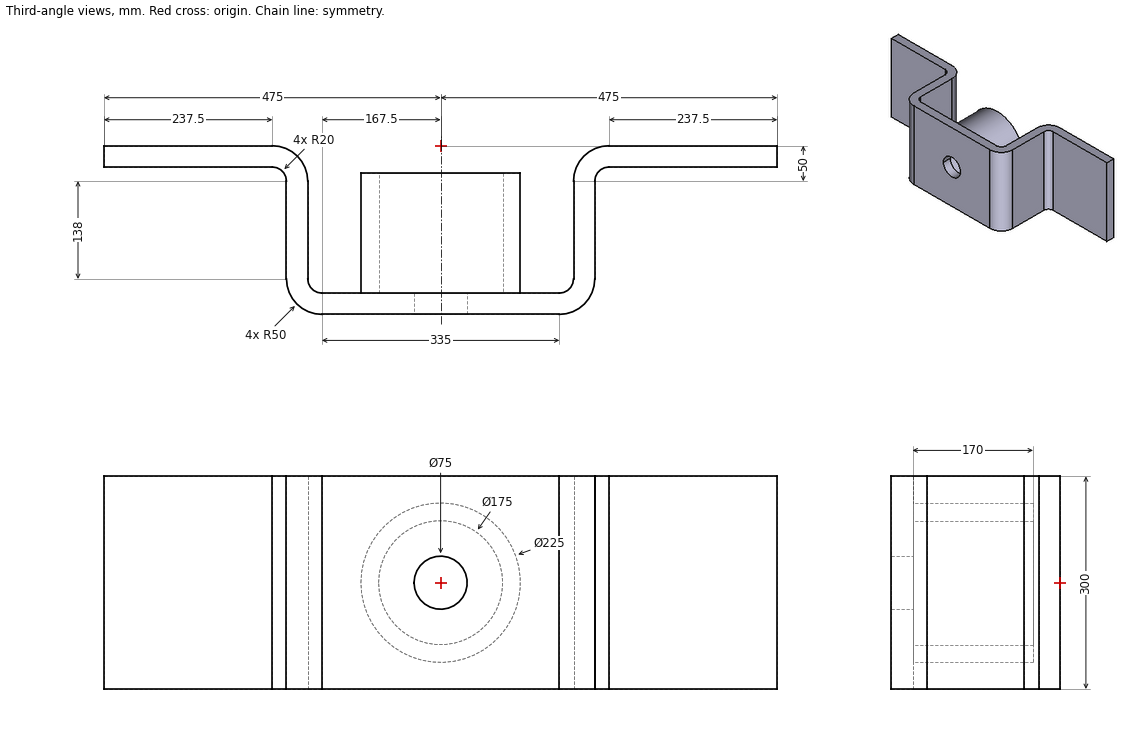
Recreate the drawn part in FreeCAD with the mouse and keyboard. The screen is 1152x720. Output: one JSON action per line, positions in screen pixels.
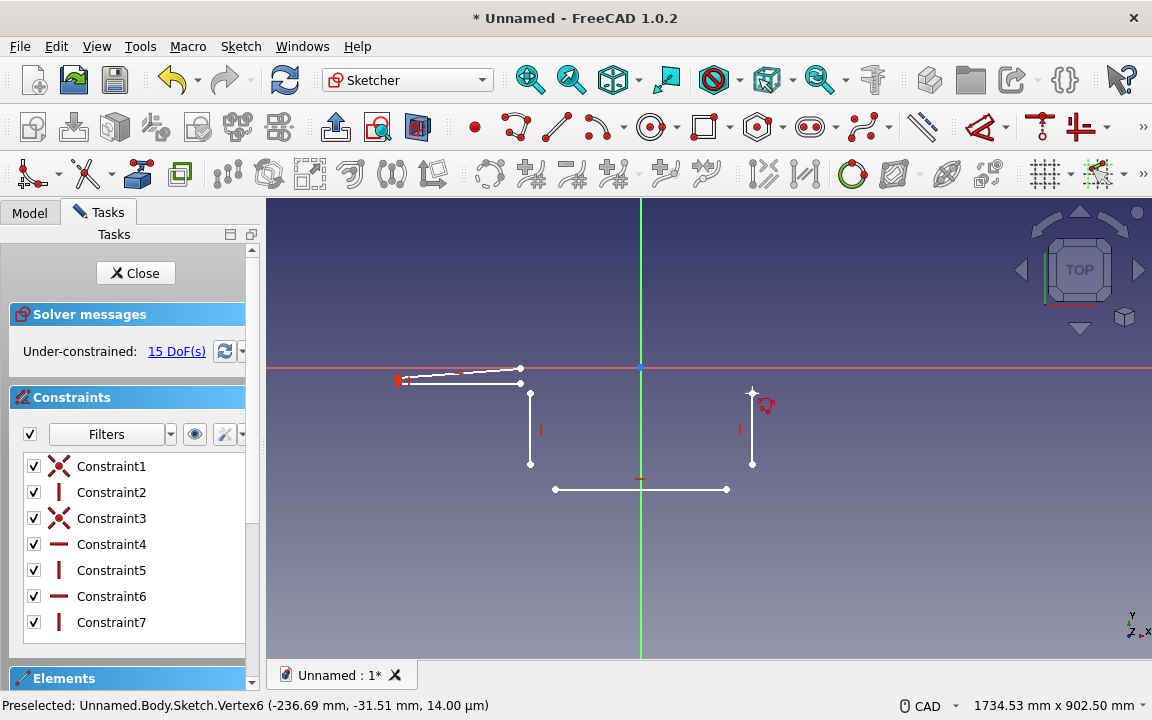
{"action": "left_click", "coordinate": [762, 383]}
{"action": "left_click", "coordinate": [884, 383]}
{"action": "left_click", "coordinate": [884, 368]}
{"action": "left_click", "coordinate": [762, 377]}
{"action": "right_click", "coordinate": [762, 377]}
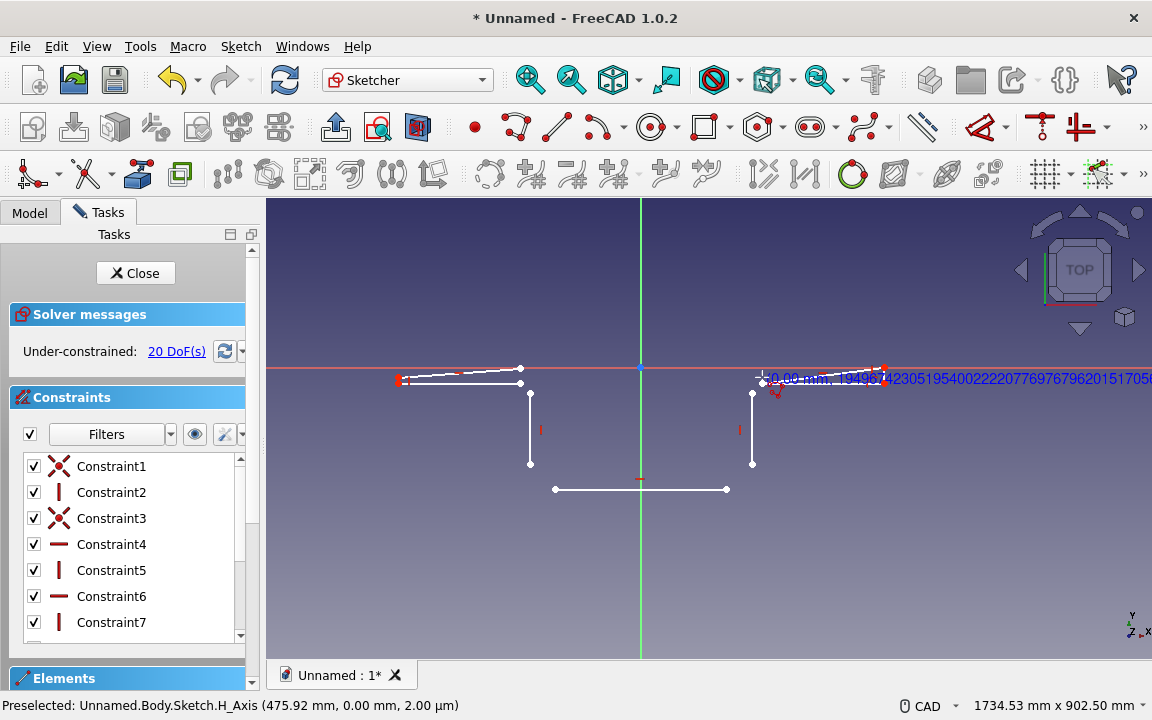
{"action": "key", "text": "g l"}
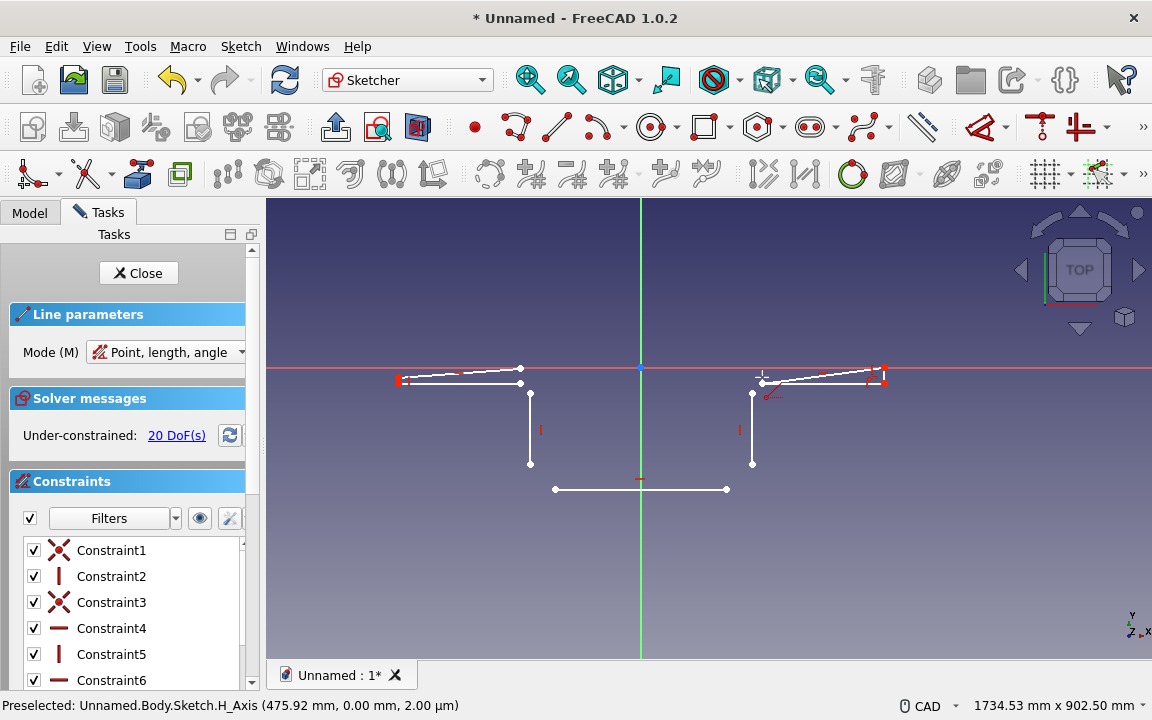
{"action": "left_click", "coordinate": [737, 393]}
{"action": "left_click", "coordinate": [737, 464]}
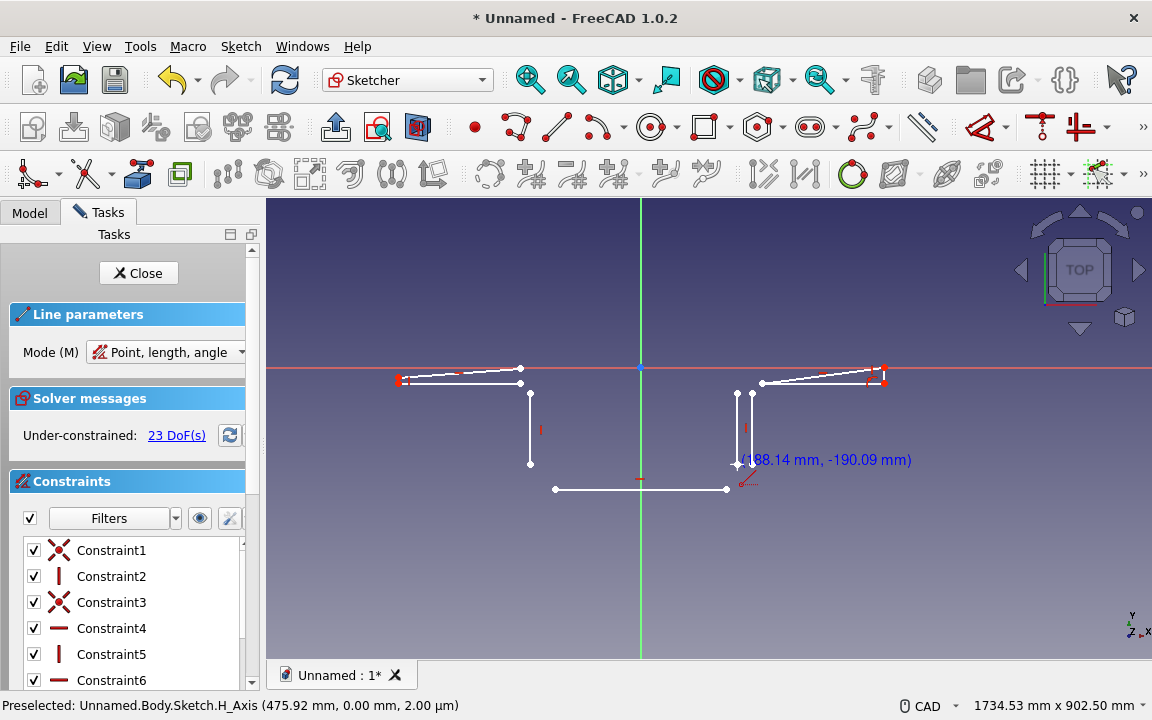
{"action": "left_click", "coordinate": [726, 474]}
{"action": "left_click", "coordinate": [555, 474]}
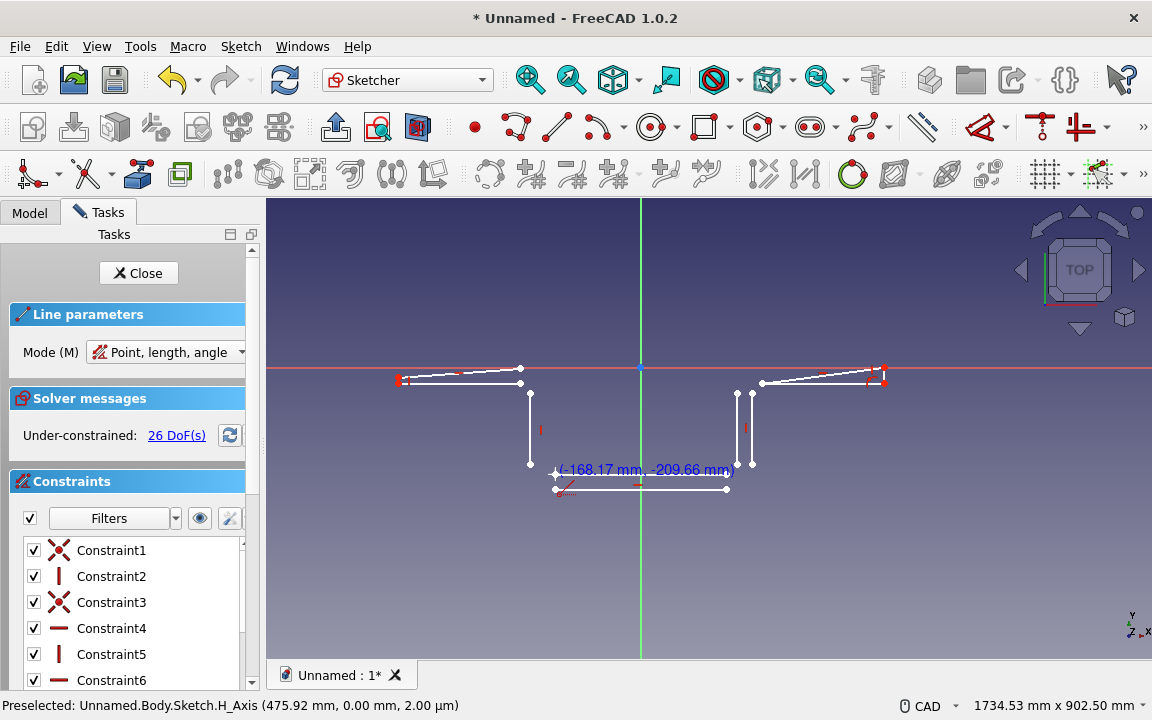
{"action": "left_click", "coordinate": [545, 464]}
{"action": "left_click", "coordinate": [545, 393]}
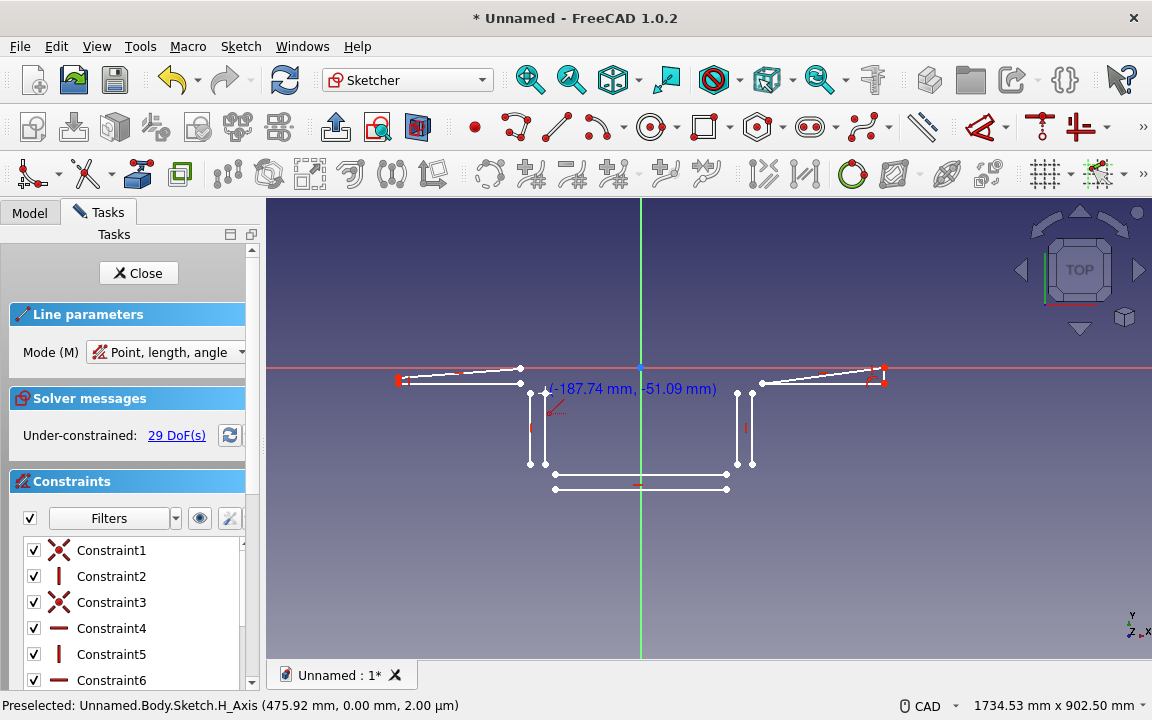
{"action": "key", "text": "g 3 a"}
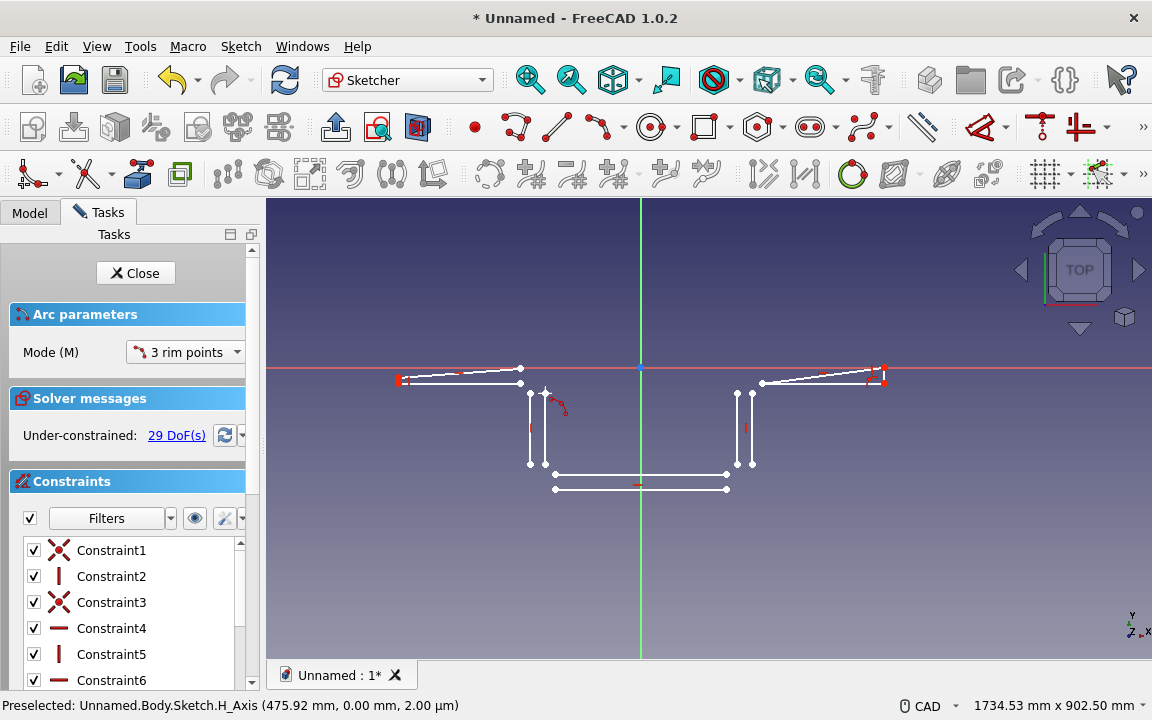
{"action": "left_click", "coordinate": [520, 384]}
{"action": "left_click", "coordinate": [530, 394]}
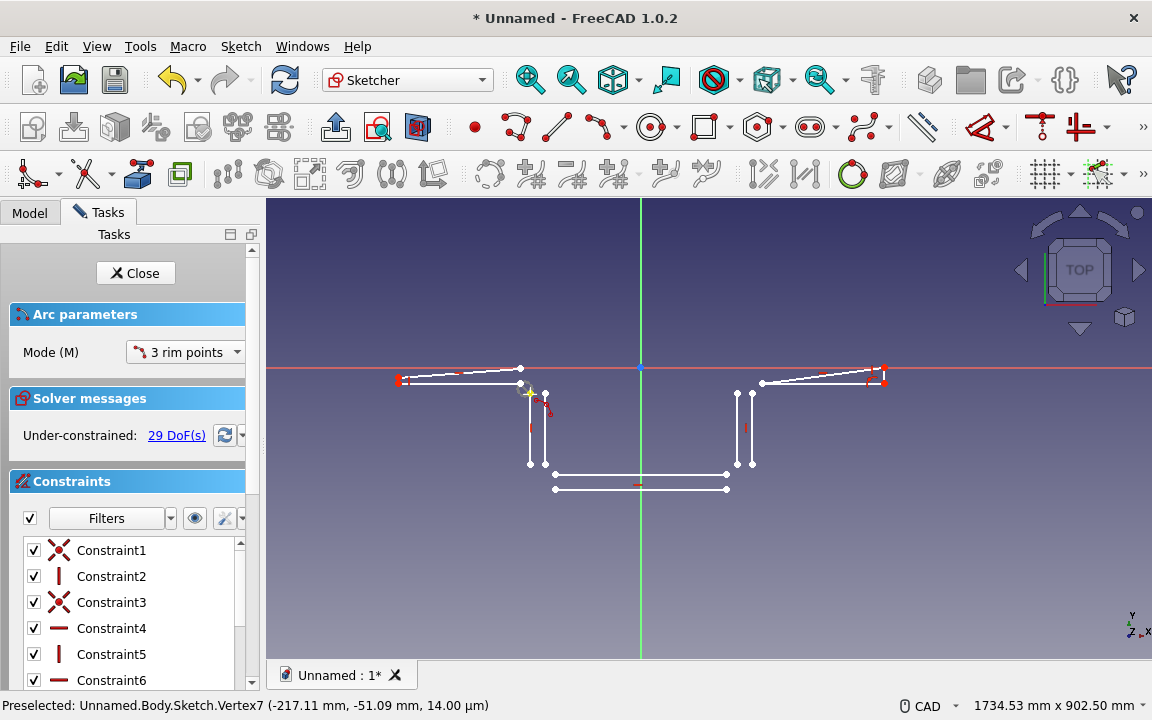
{"action": "scroll", "coordinate": [527, 386], "scroll_direction": "up", "scroll_amount": 9}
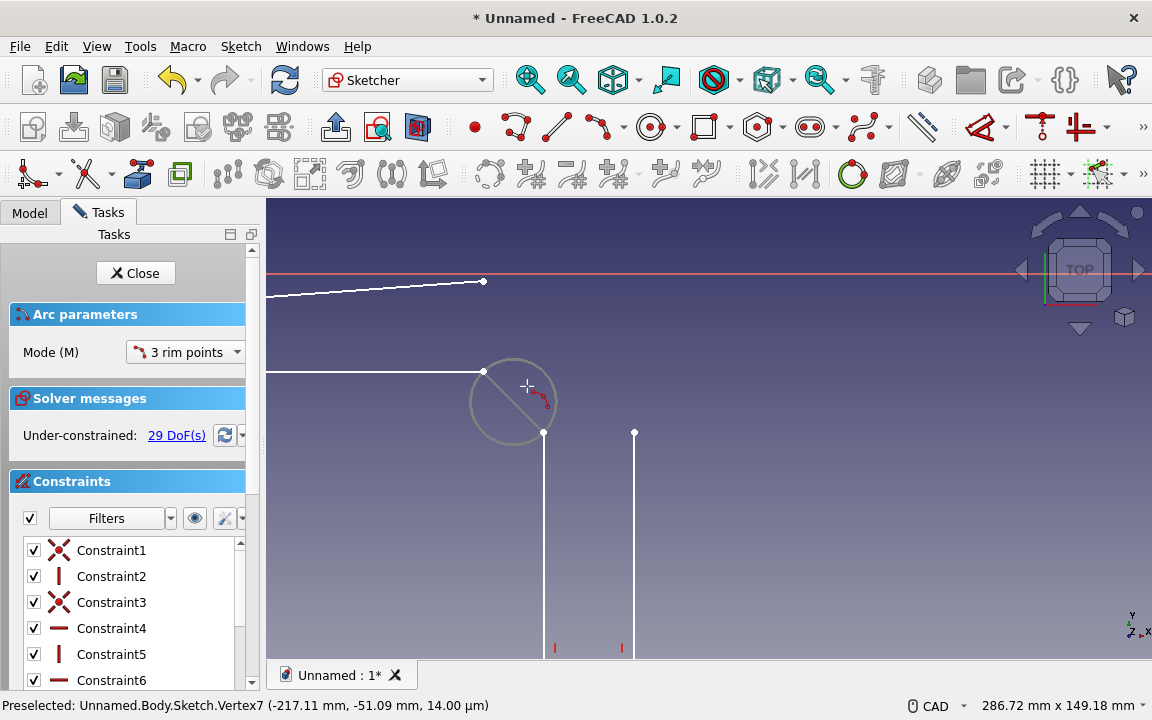
{"action": "left_click", "coordinate": [524, 385]}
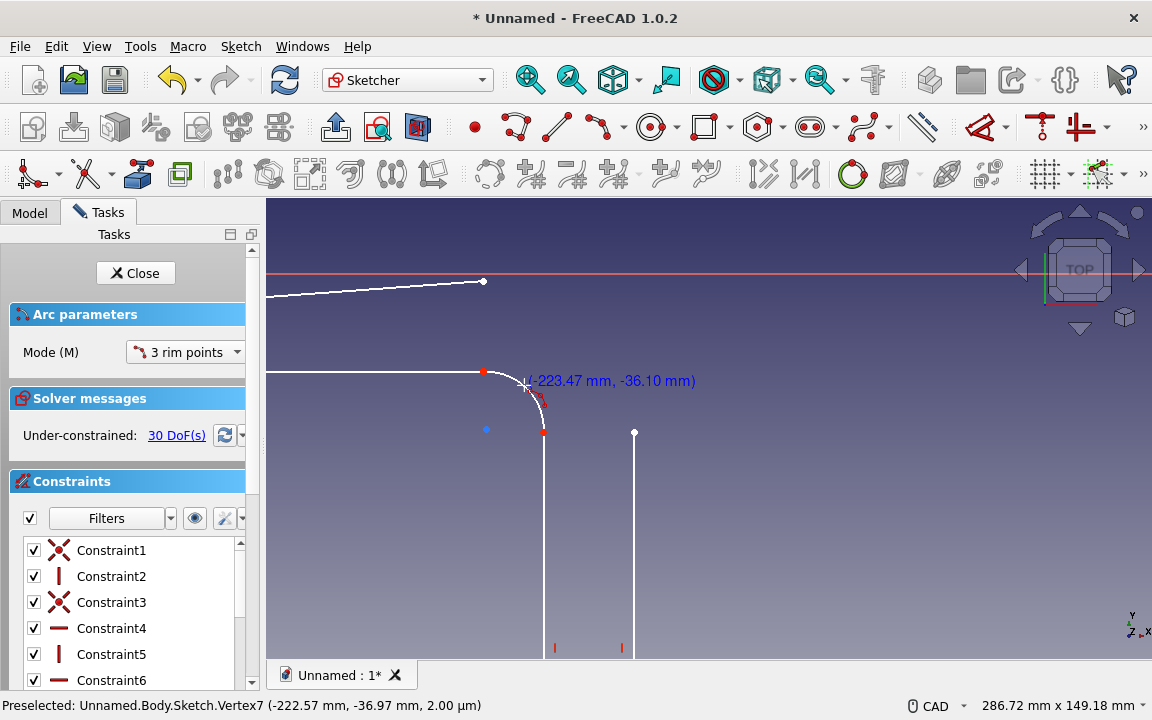
{"action": "scroll", "coordinate": [527, 386], "scroll_direction": "down", "scroll_amount": 9}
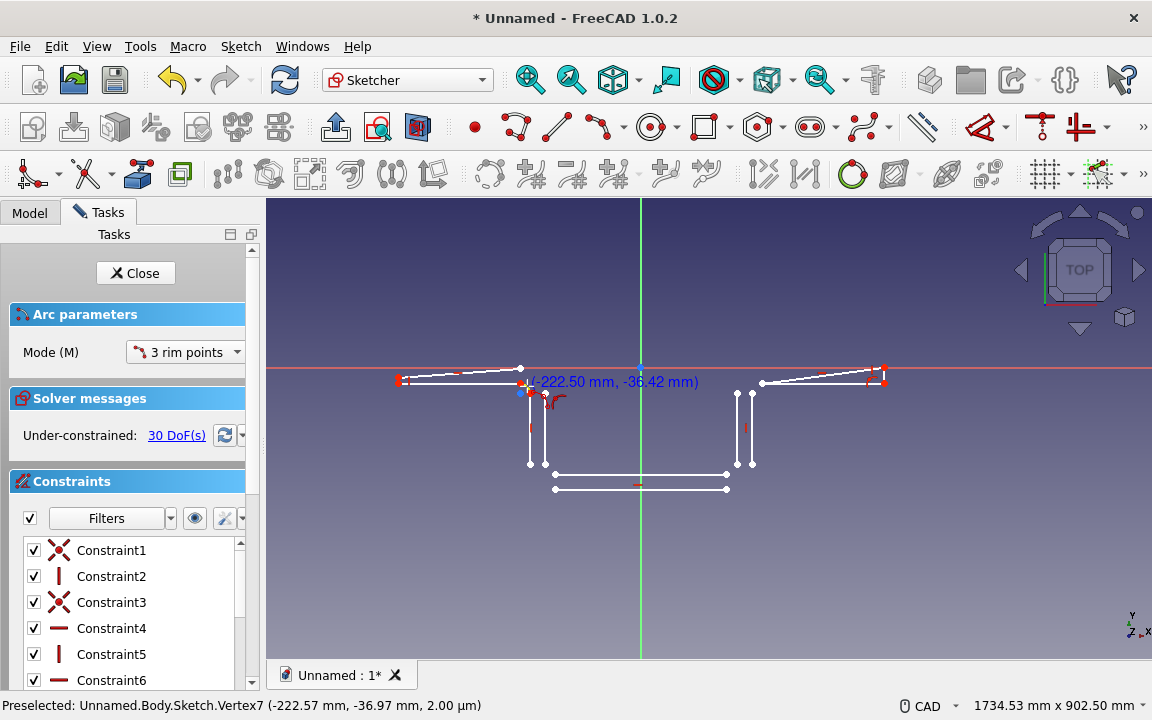
{"action": "left_click", "coordinate": [530, 465]}
{"action": "left_click", "coordinate": [555, 490]}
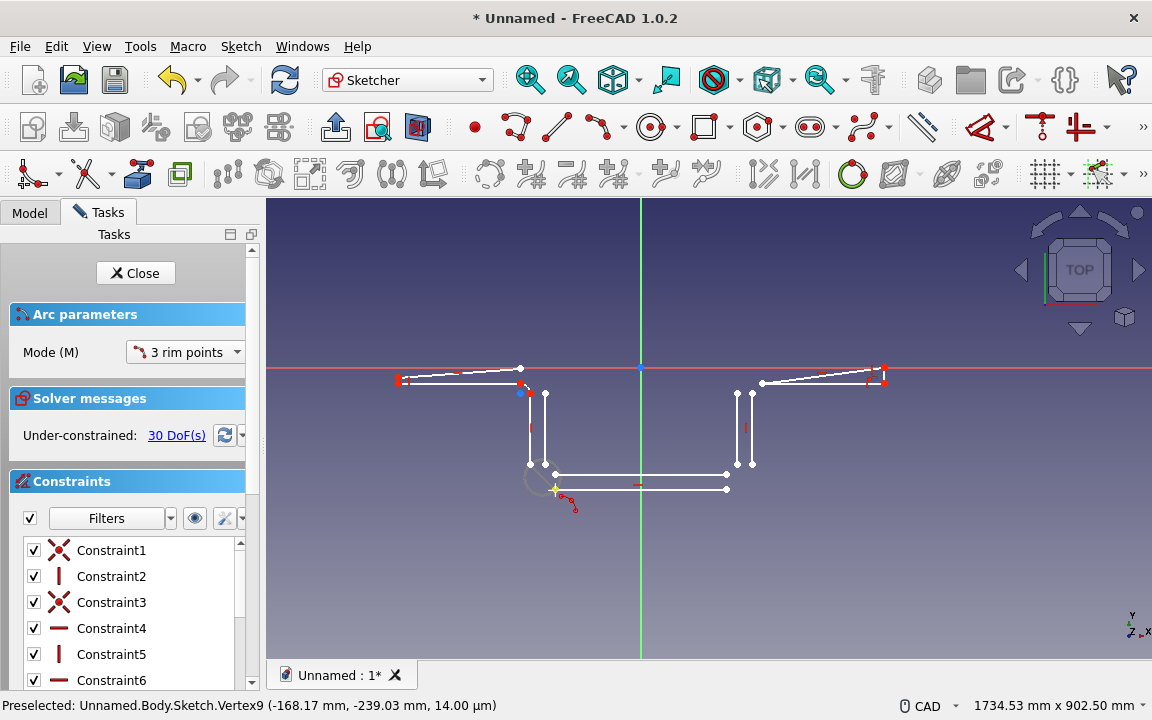
{"action": "scroll", "coordinate": [537, 482], "scroll_direction": "up", "scroll_amount": 4}